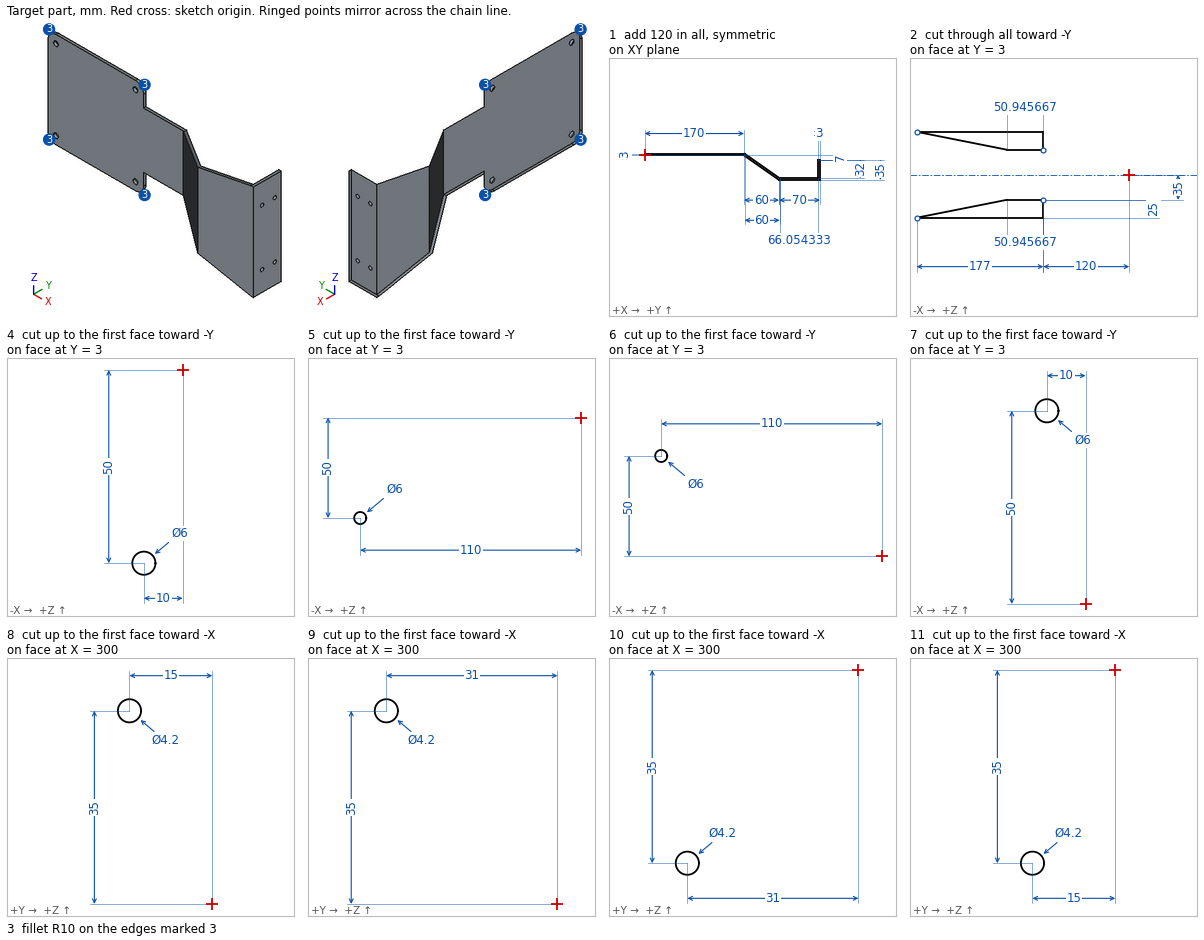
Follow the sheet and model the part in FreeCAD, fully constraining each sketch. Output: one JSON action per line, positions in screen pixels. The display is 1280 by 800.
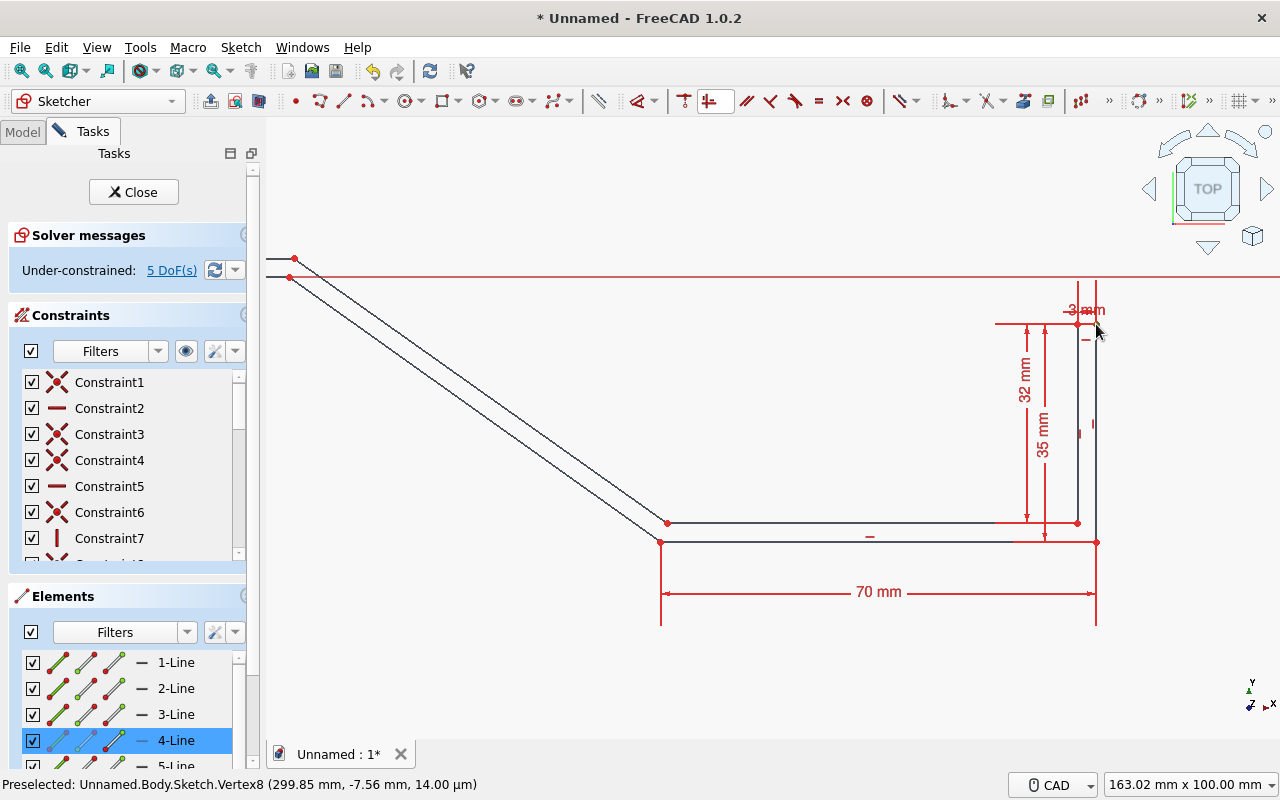
{"action": "left_click", "coordinate": [656, 102]}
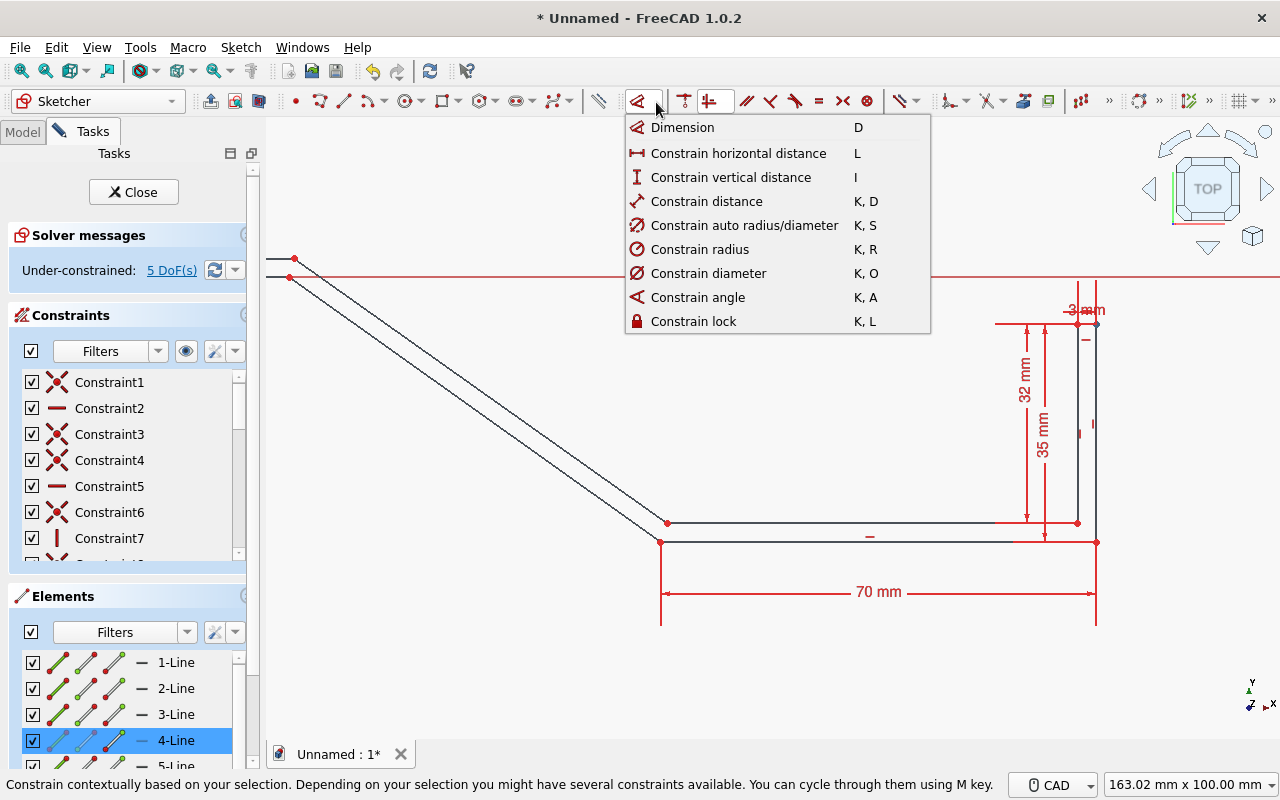
{"action": "left_click", "coordinate": [778, 177]}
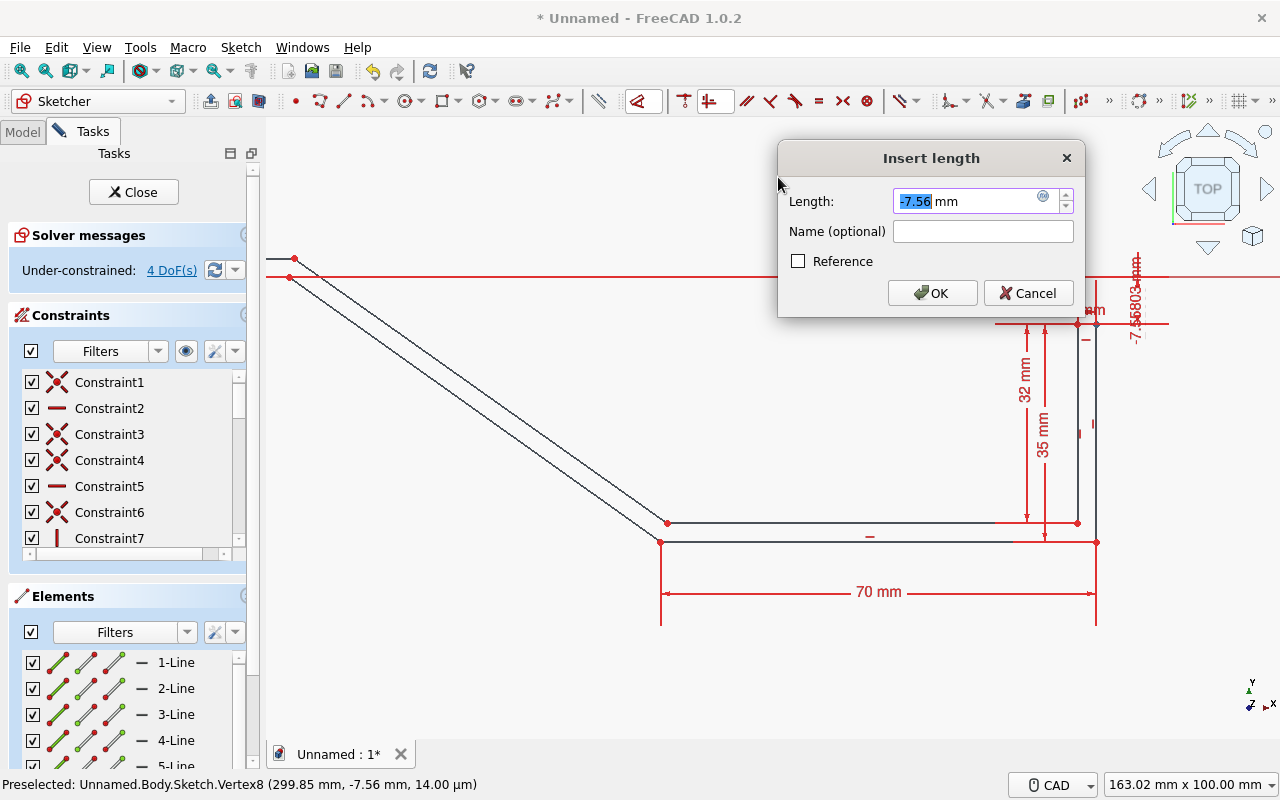
{"action": "type", "text": "-7"}
{"action": "key", "text": "Return"}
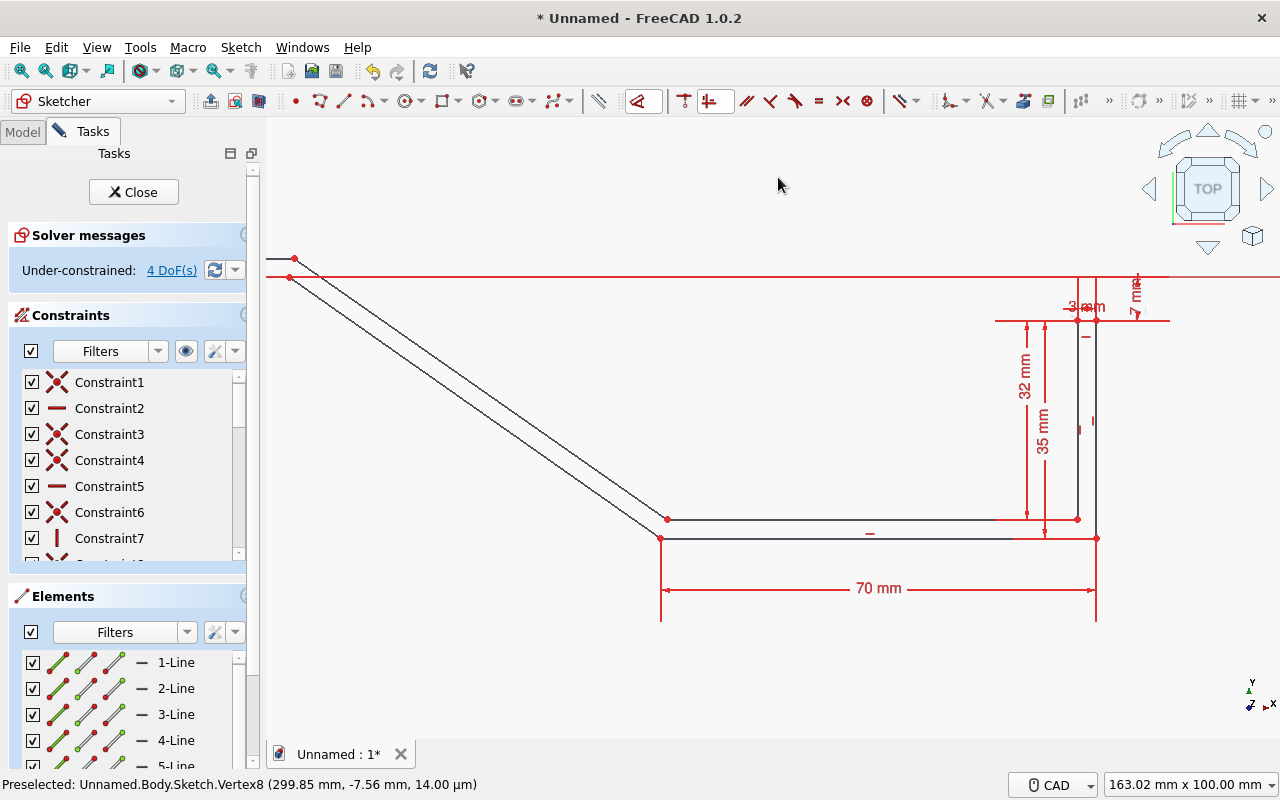
{"action": "scroll", "coordinate": [937, 441], "scroll_direction": "down", "scroll_amount": 6}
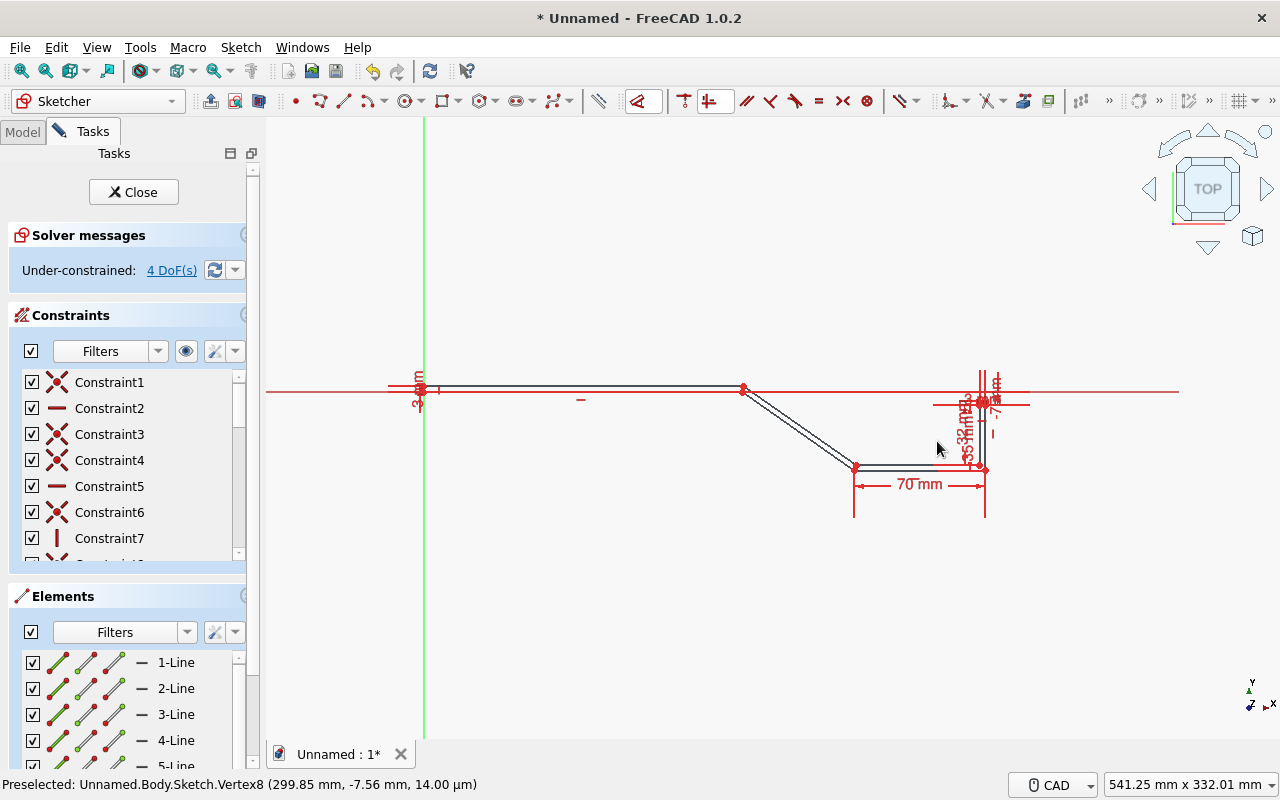
{"action": "scroll", "coordinate": [519, 392], "scroll_direction": "up", "scroll_amount": 5}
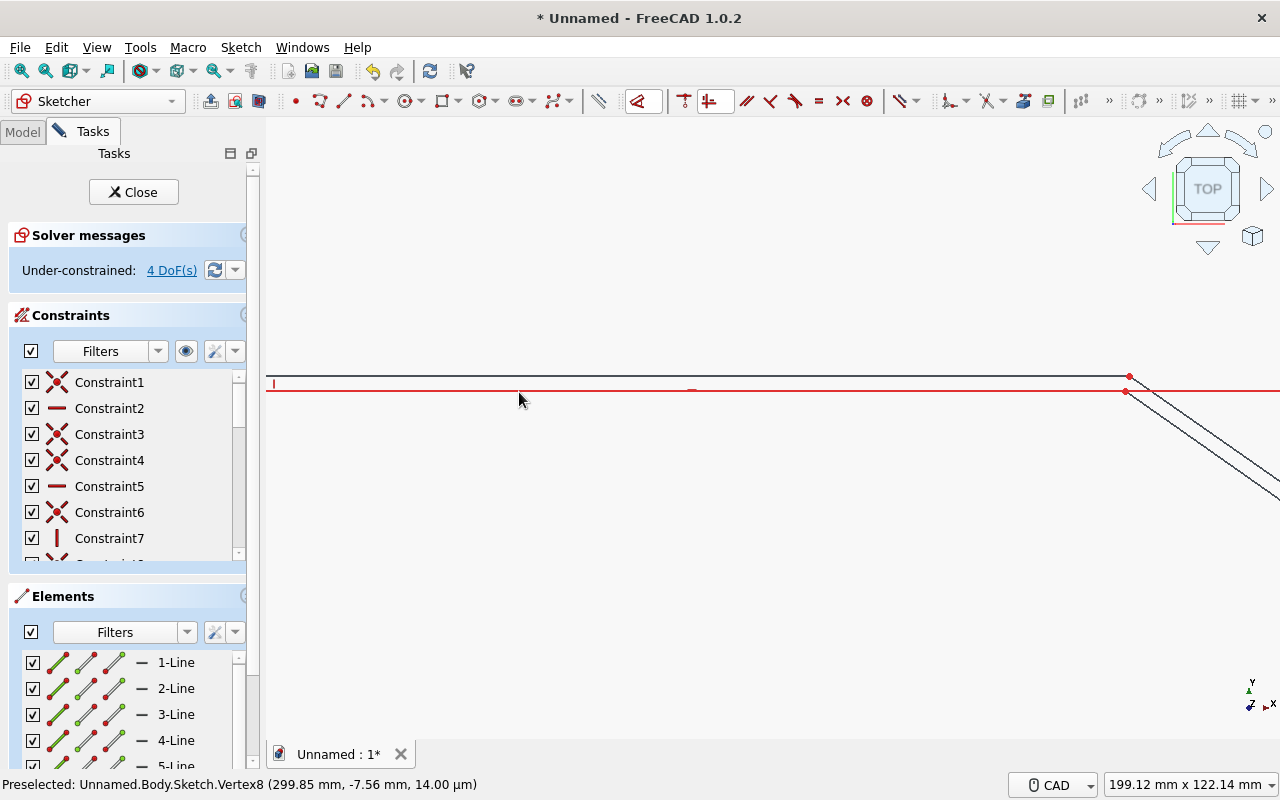
{"action": "left_click", "coordinate": [519, 391]}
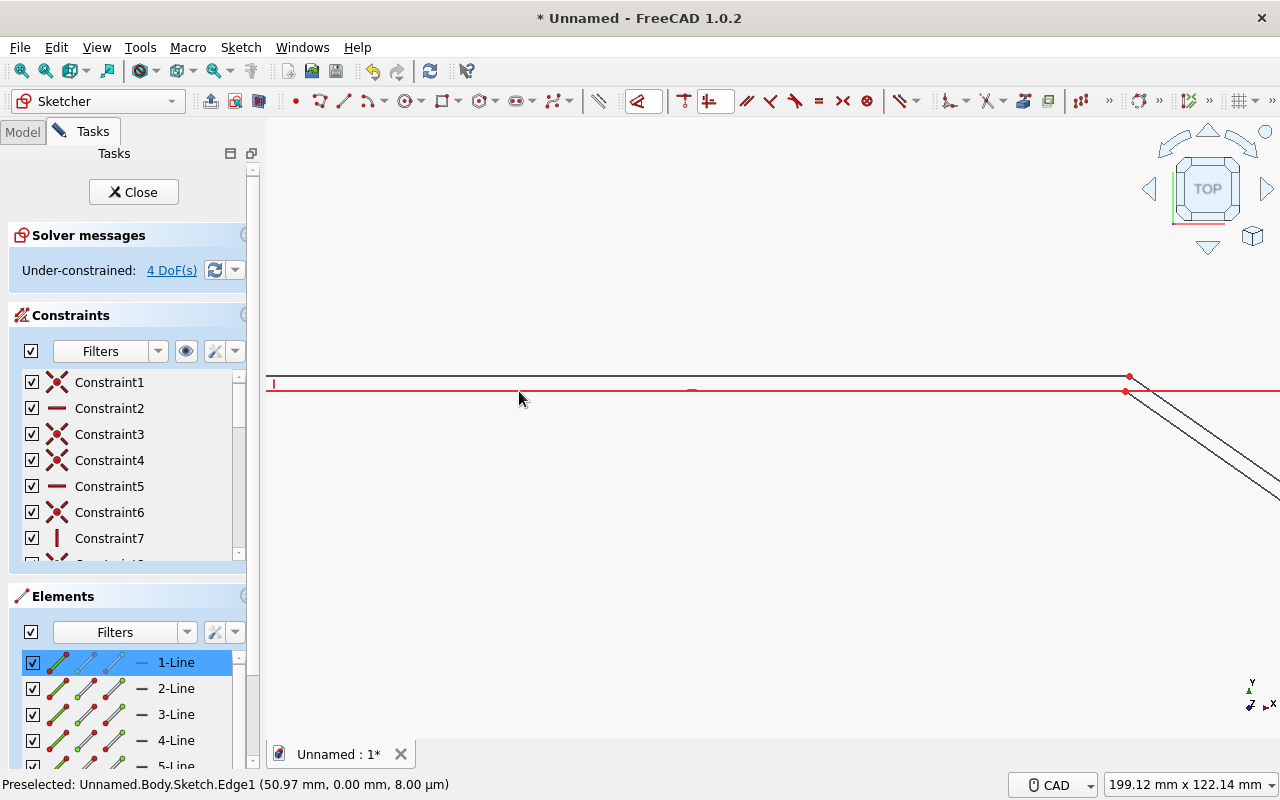
{"action": "key", "text": "l"}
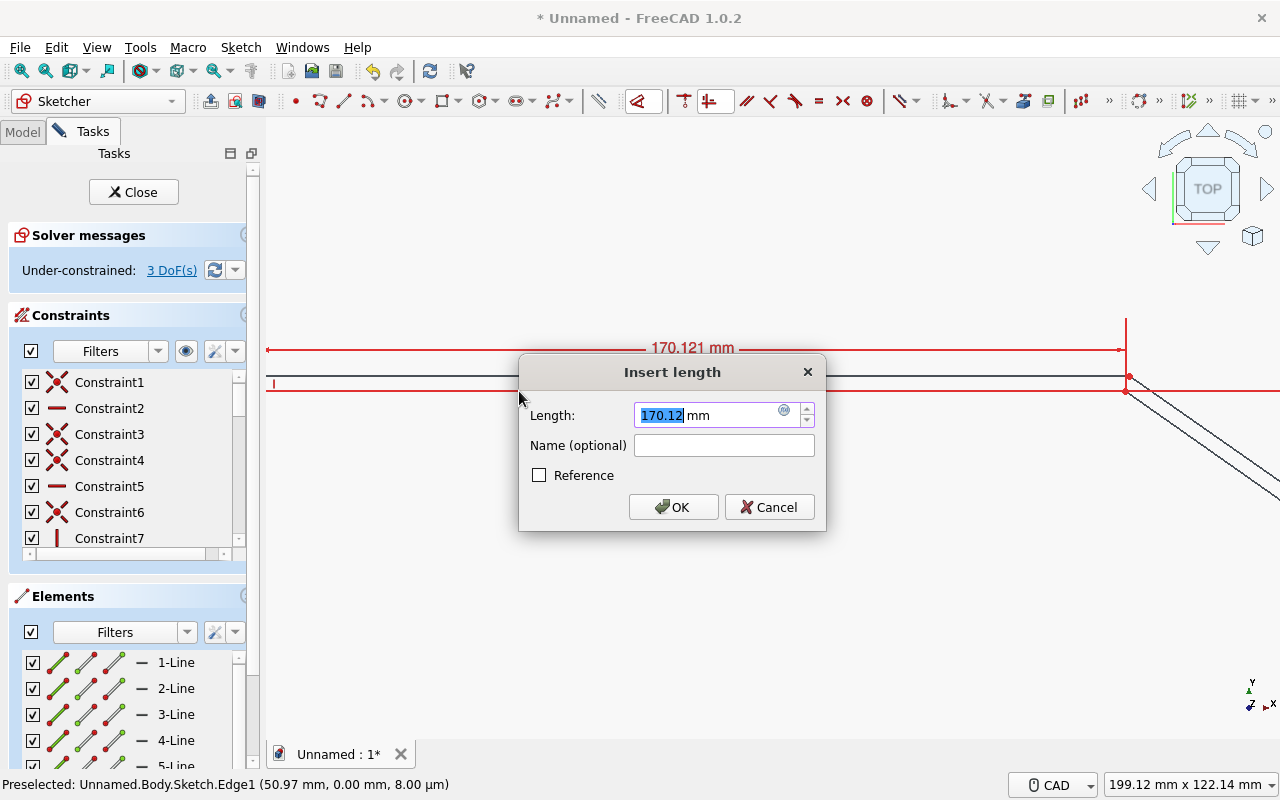
{"action": "type", "text": "170"}
{"action": "key", "text": "Return"}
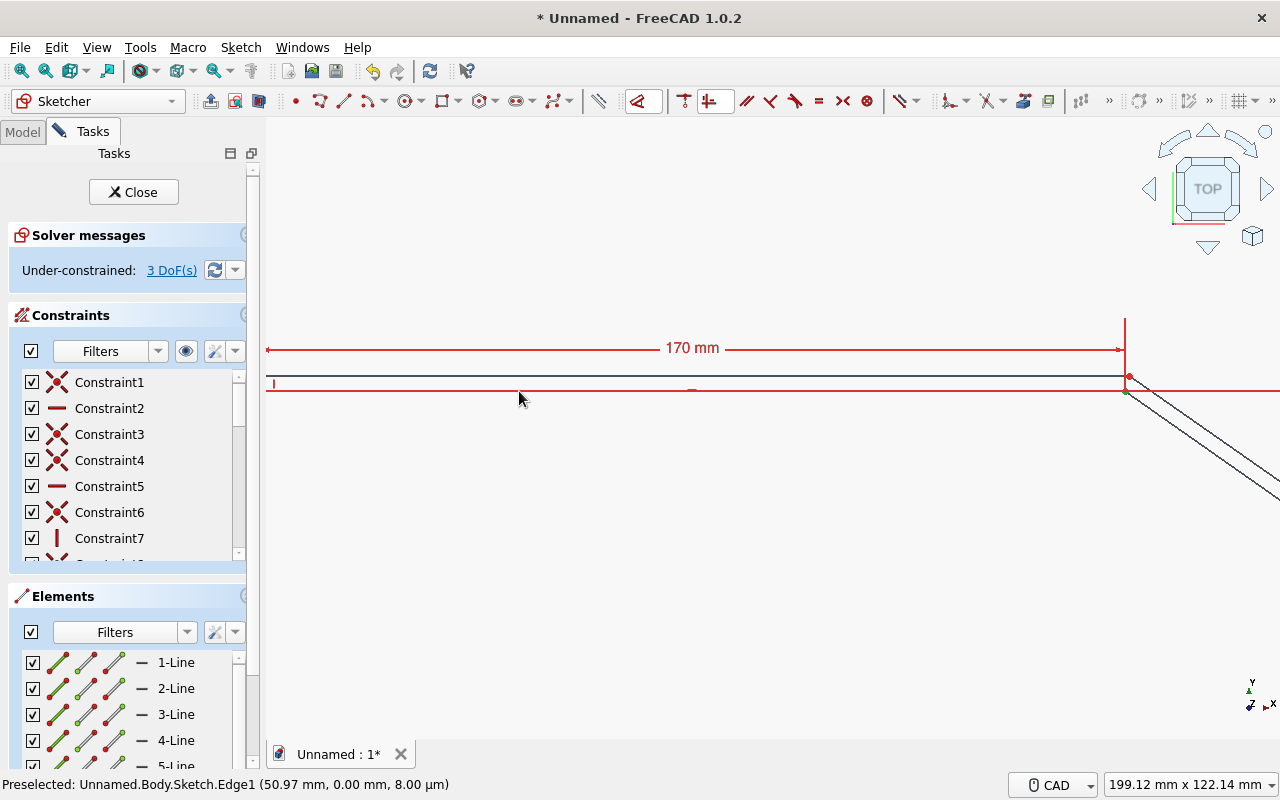
{"action": "scroll", "coordinate": [519, 391], "scroll_direction": "down", "scroll_amount": 5}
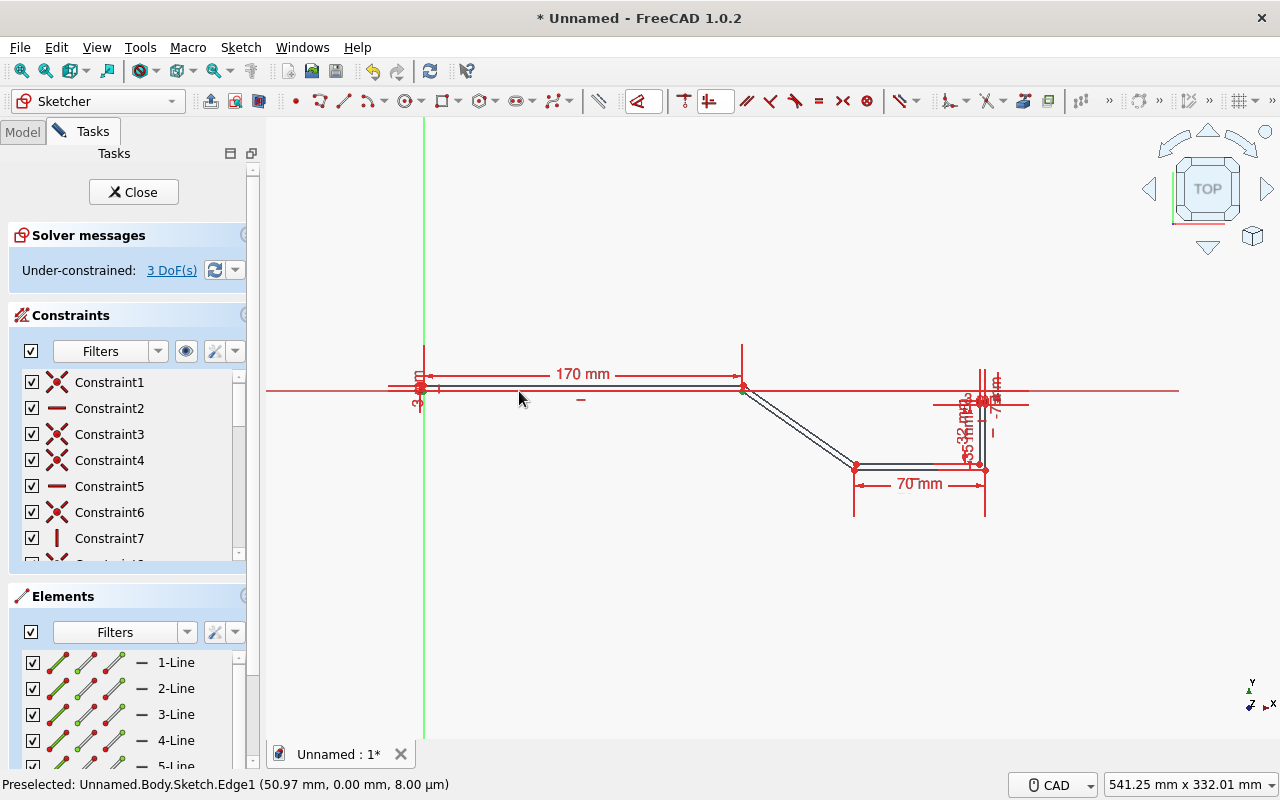
{"action": "scroll", "coordinate": [776, 415], "scroll_direction": "up", "scroll_amount": 5}